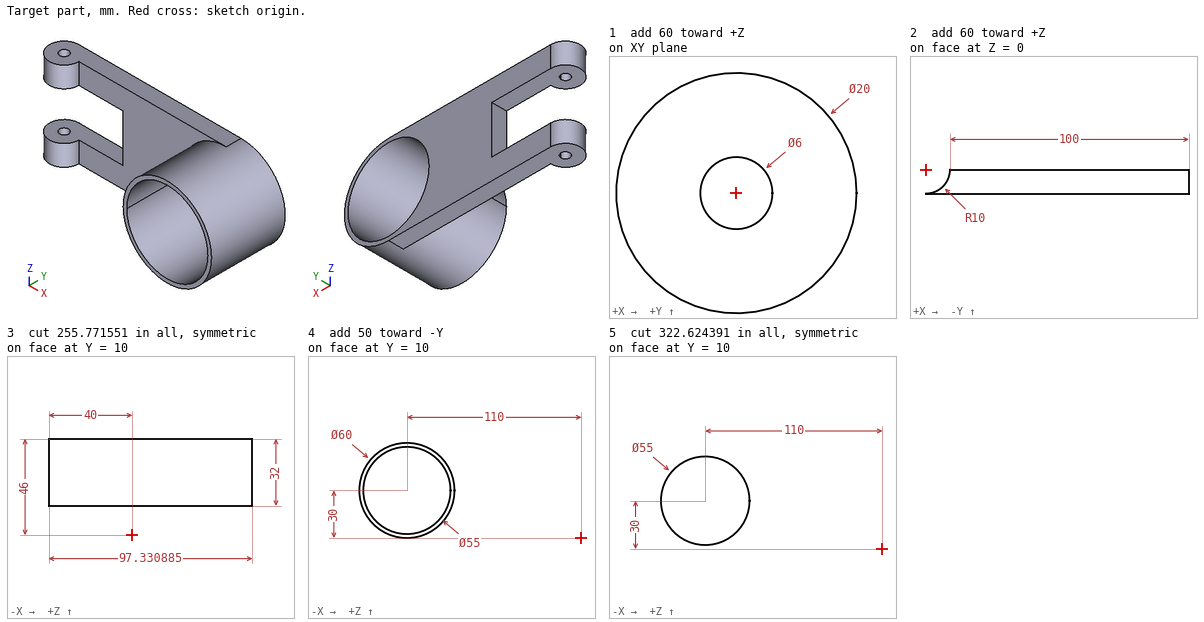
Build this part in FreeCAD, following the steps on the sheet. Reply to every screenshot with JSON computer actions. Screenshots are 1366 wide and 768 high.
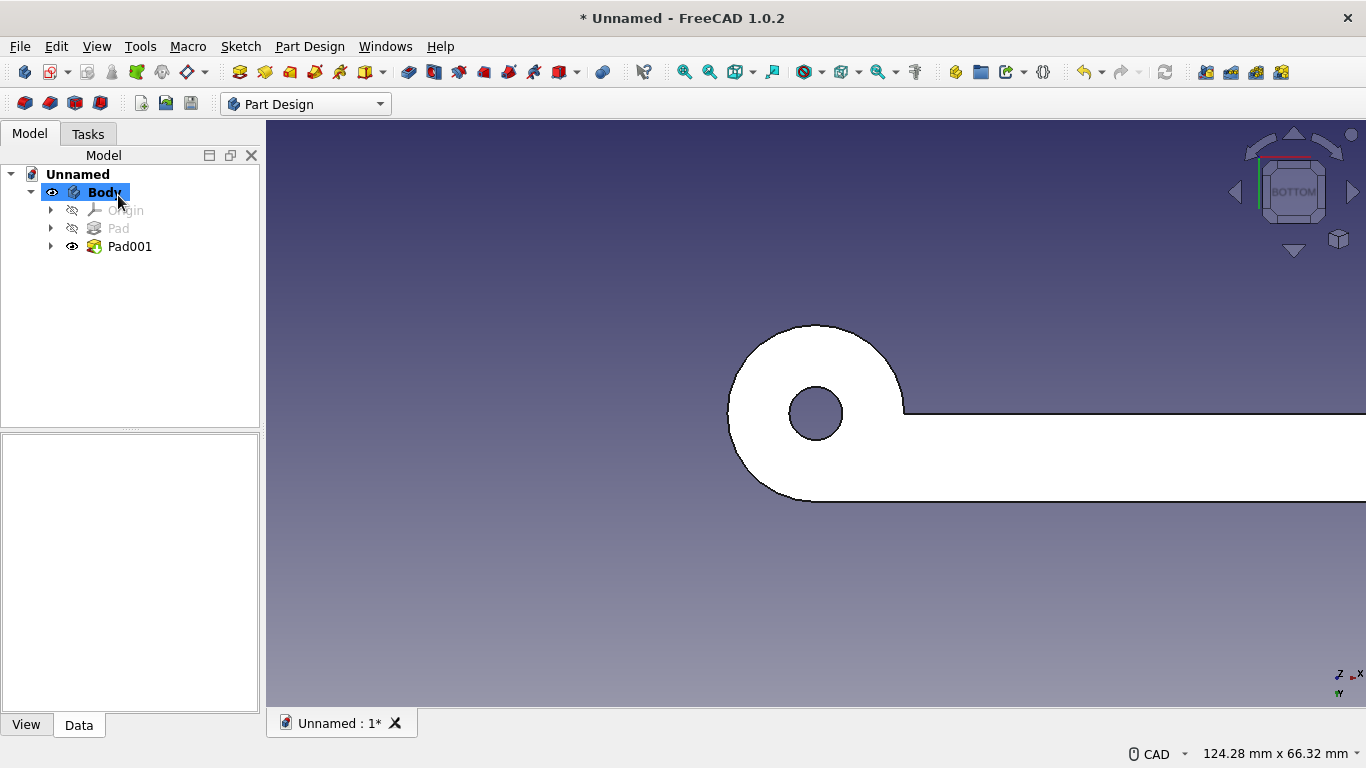
{"action": "left_click", "coordinate": [685, 72]}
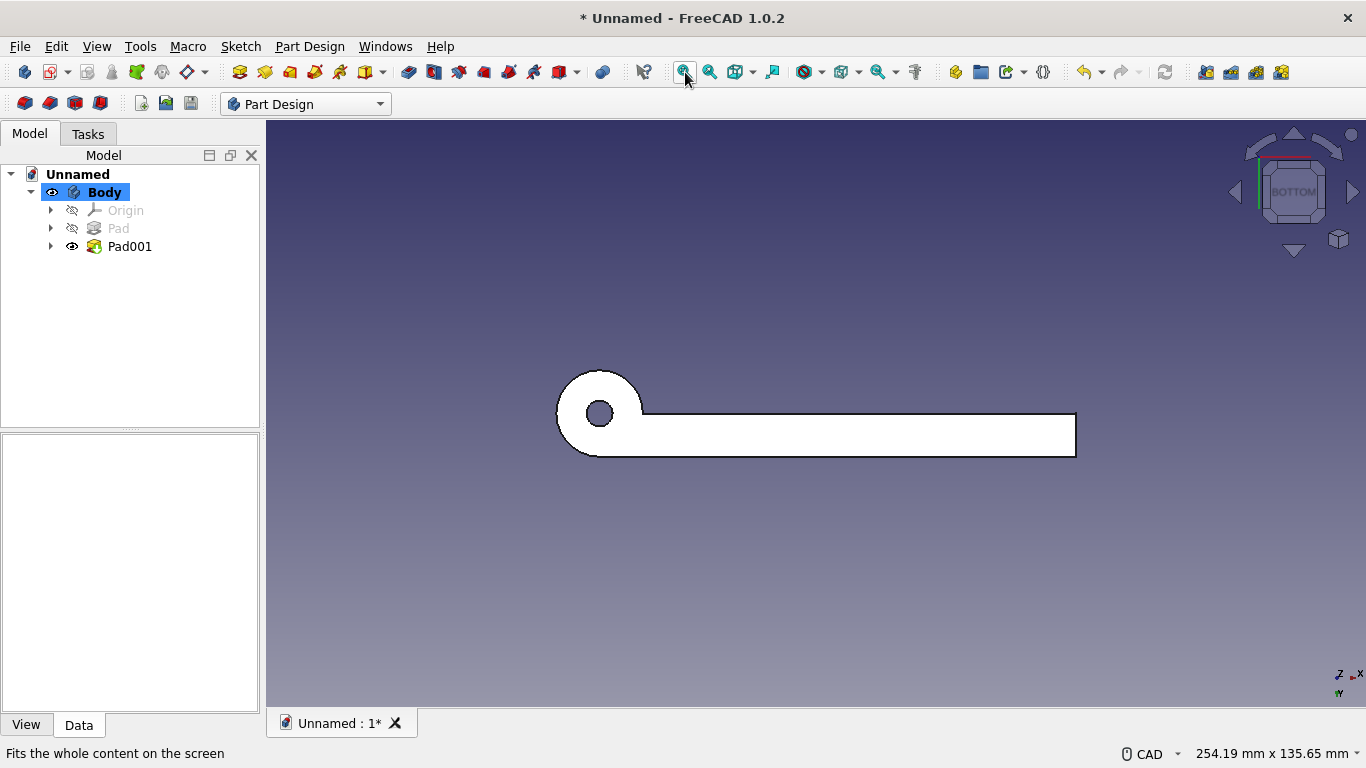
{"action": "key", "text": "4"}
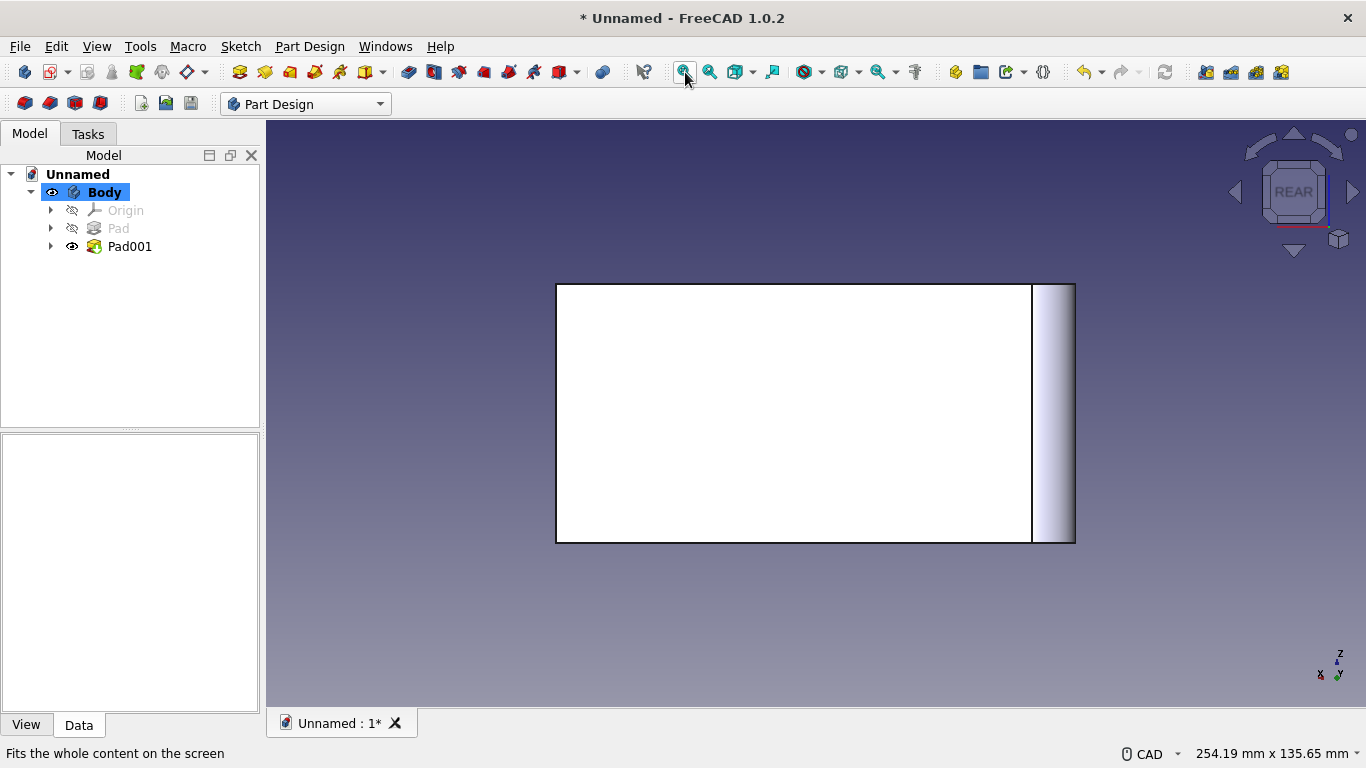
{"action": "left_click", "coordinate": [726, 412]}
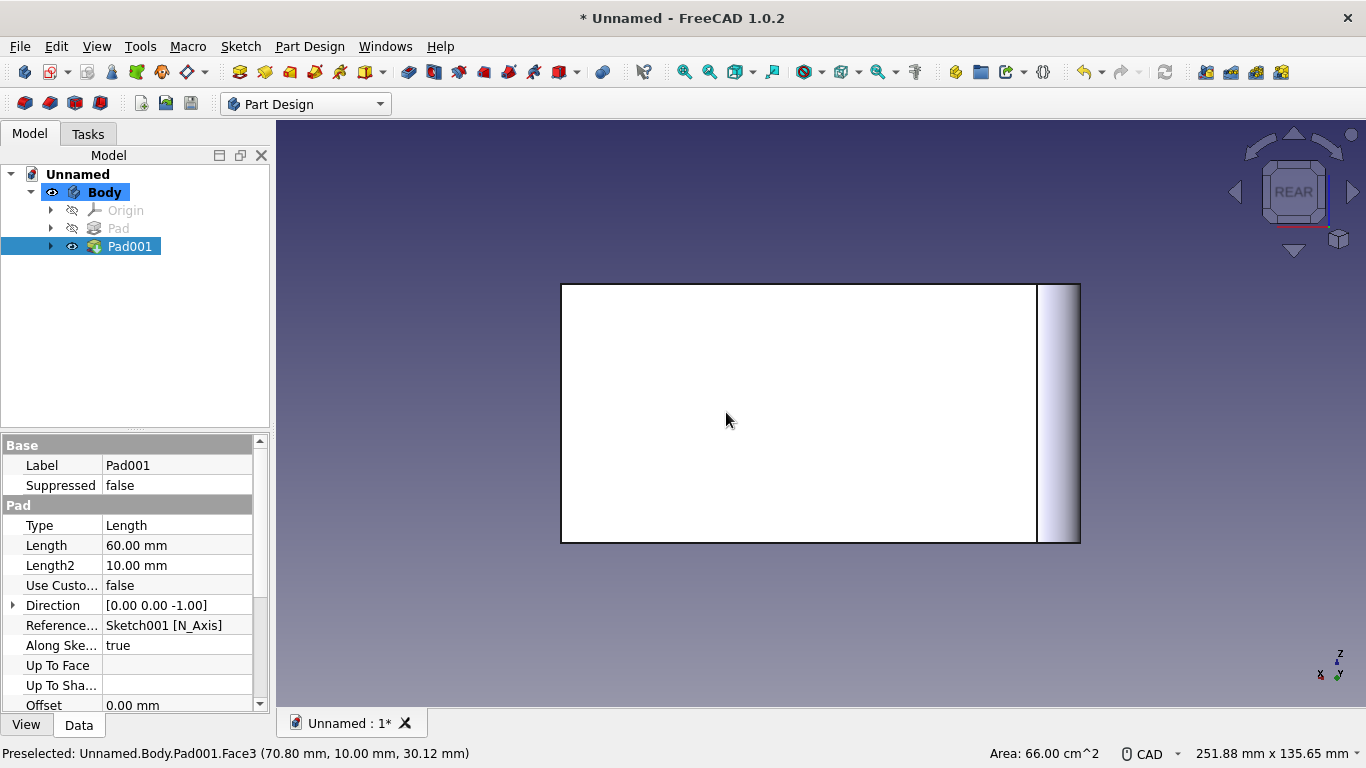
{"action": "left_click", "coordinate": [50, 72]}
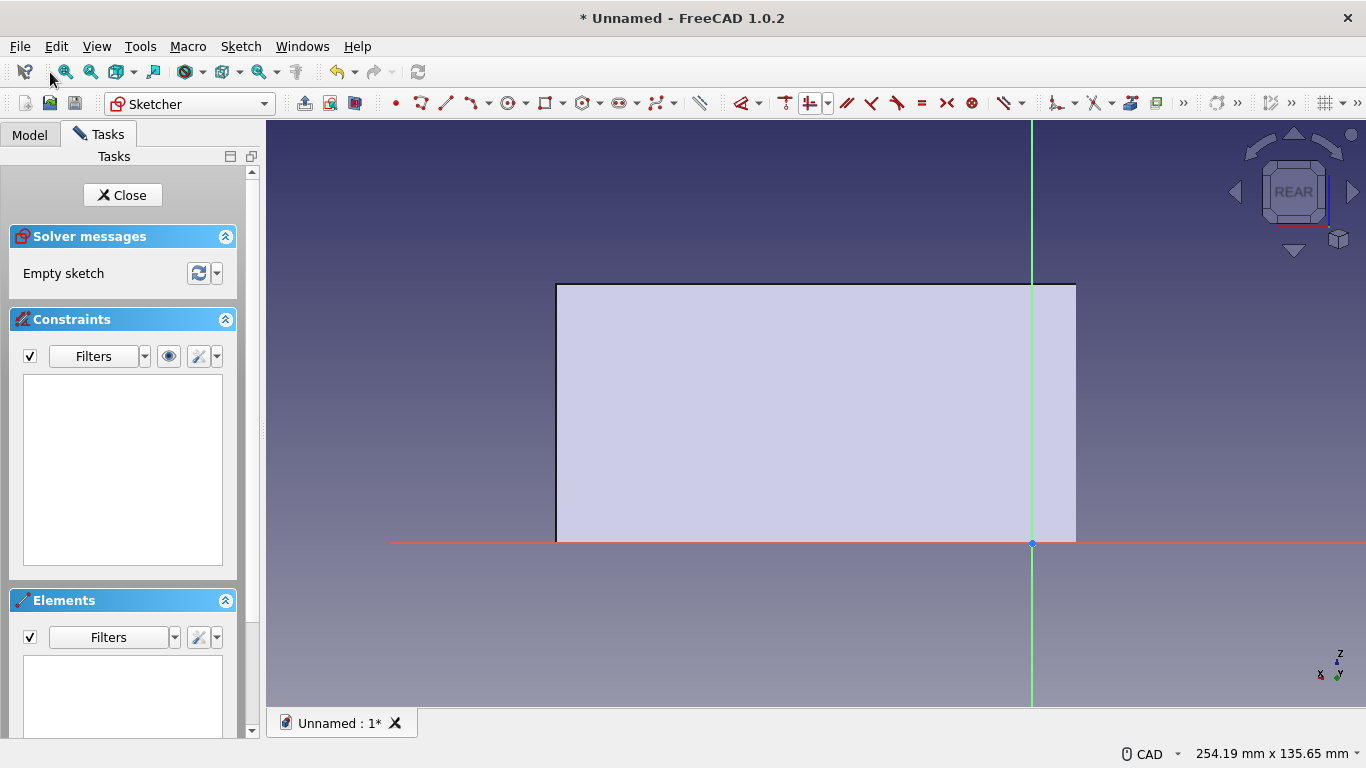
{"action": "scroll", "coordinate": [294, 277], "scroll_direction": "down", "scroll_amount": 1}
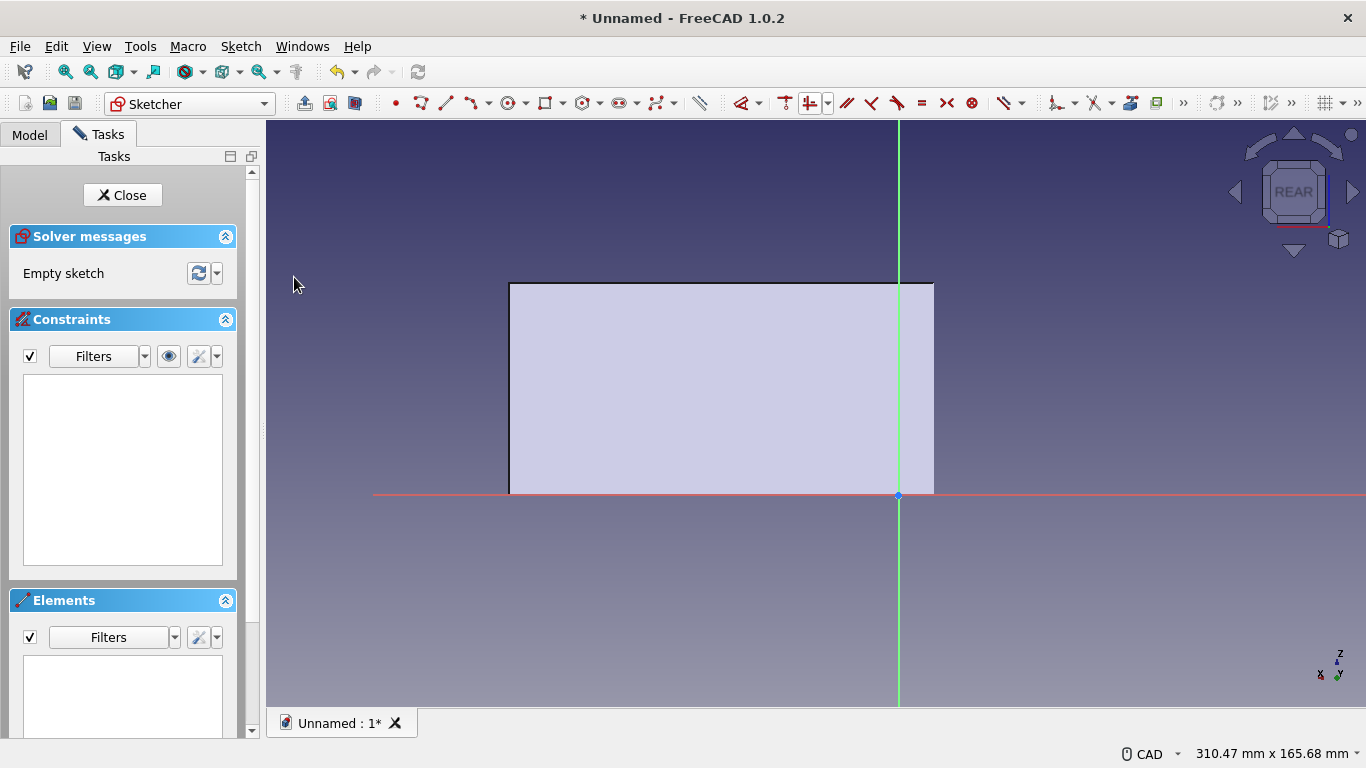
{"action": "scroll", "coordinate": [1150, 414], "scroll_direction": "up", "scroll_amount": 3}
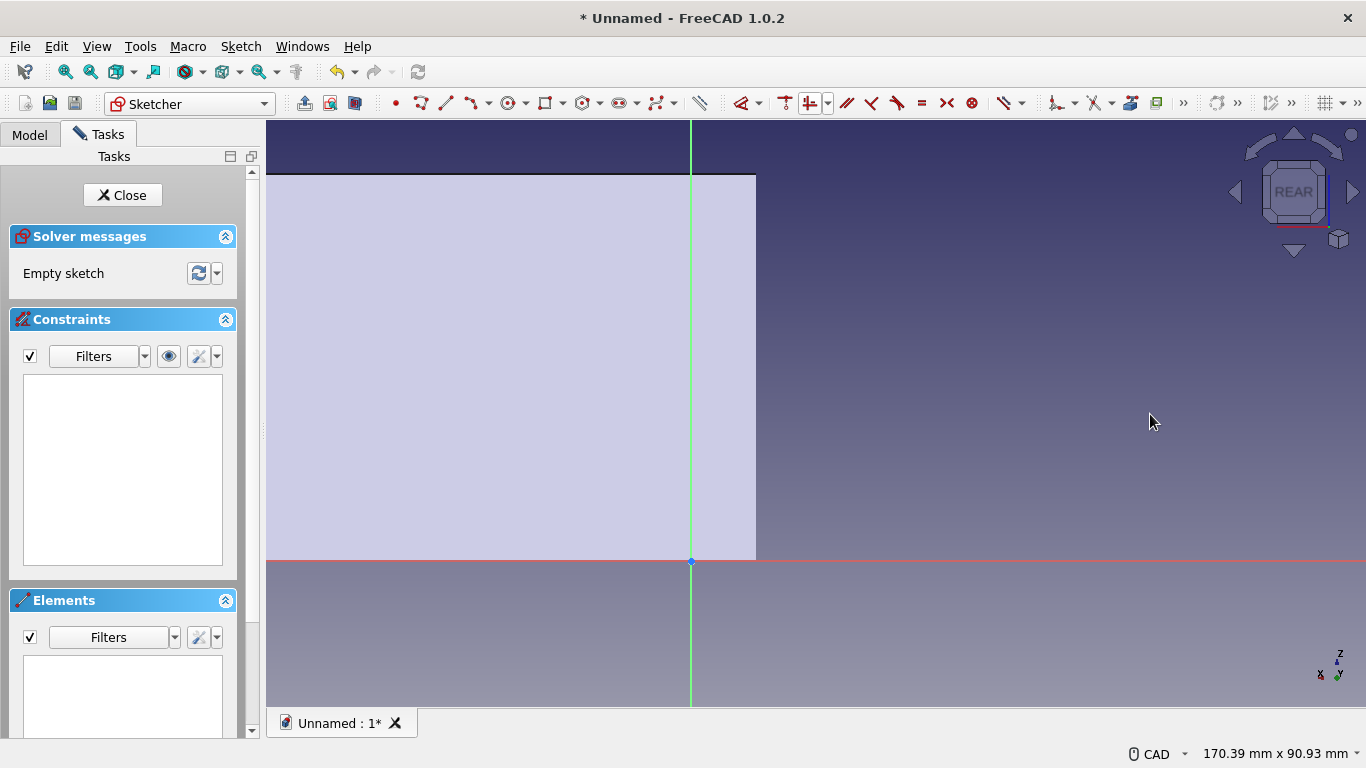
{"action": "left_click", "coordinate": [544, 104]}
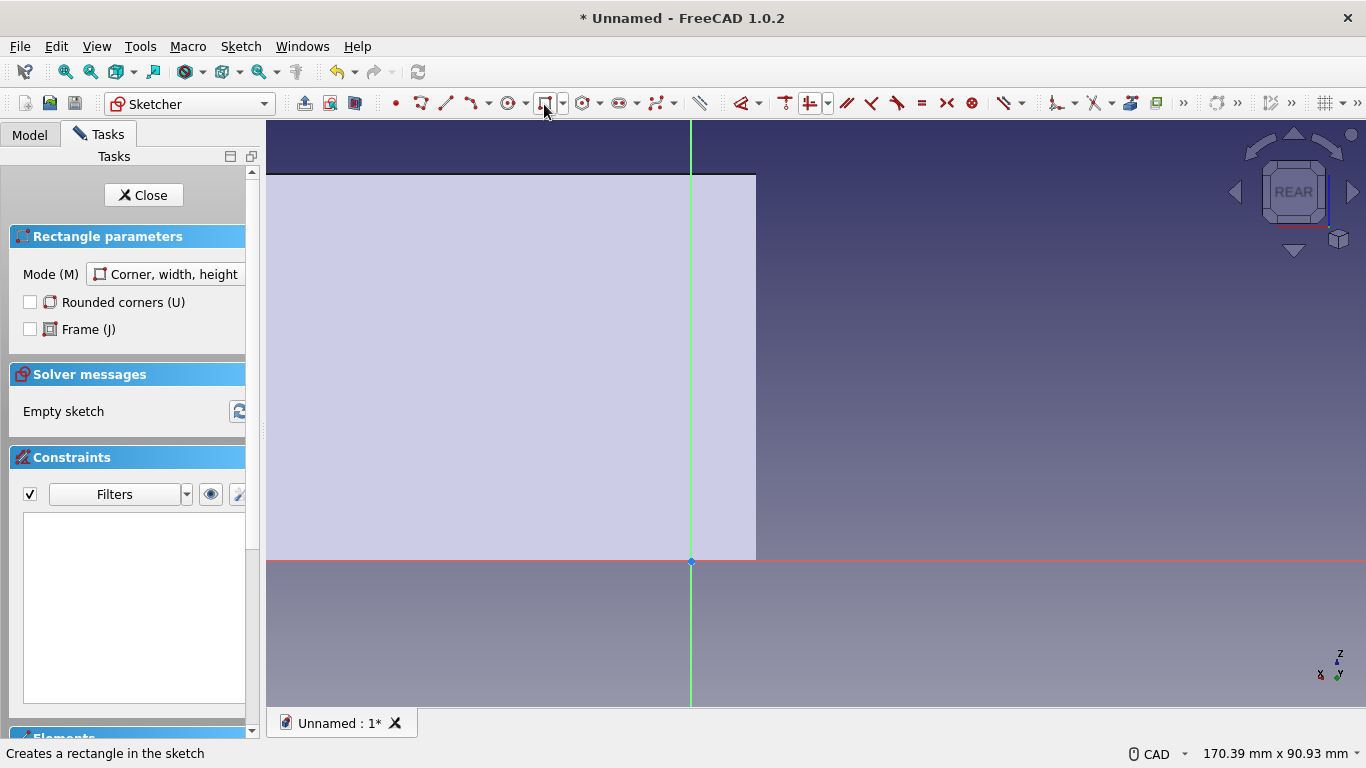
{"action": "left_click", "coordinate": [433, 264]}
{"action": "mouse_move", "coordinate": [1061, 471]}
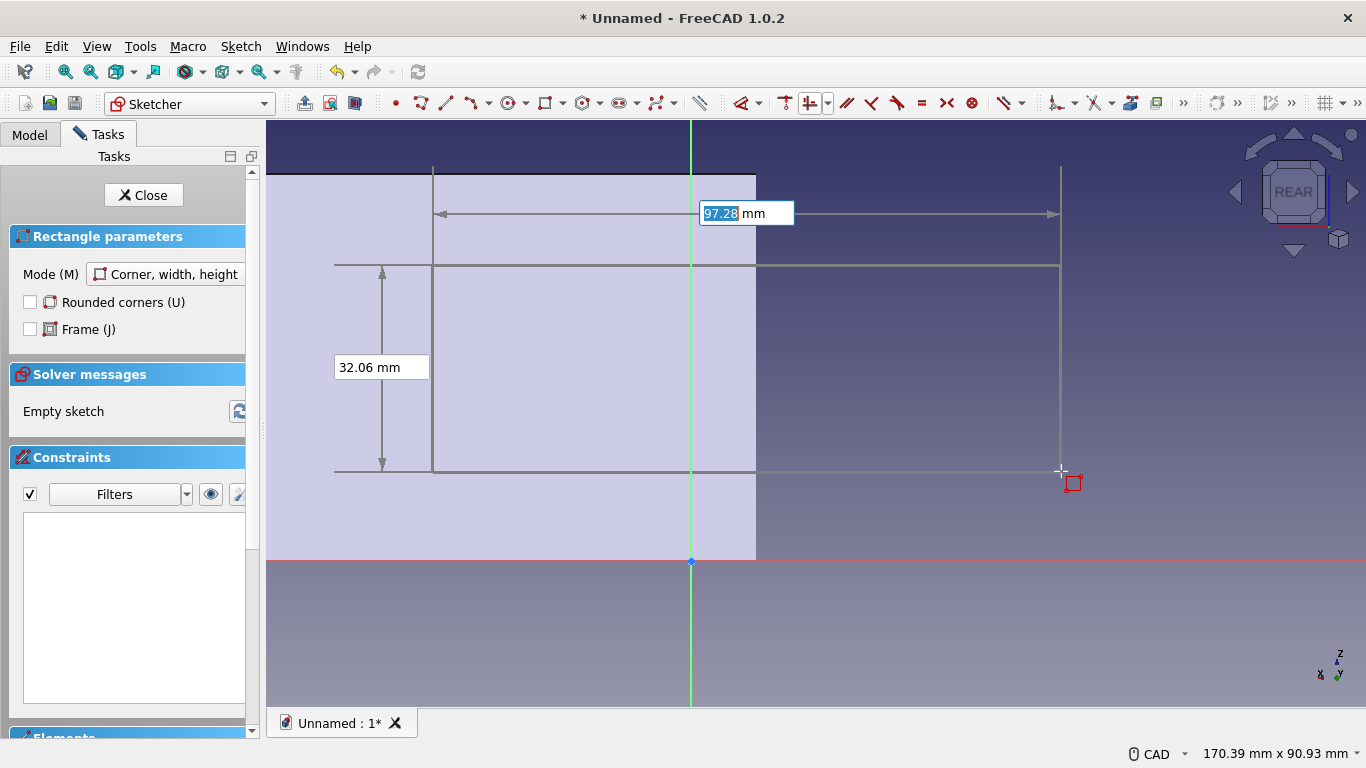
{"action": "type", "text": "97.330885"}
{"action": "key", "text": "Tab"}
{"action": "type", "text": "32"}
{"action": "key", "text": "Return"}
{"action": "key", "text": "Escape"}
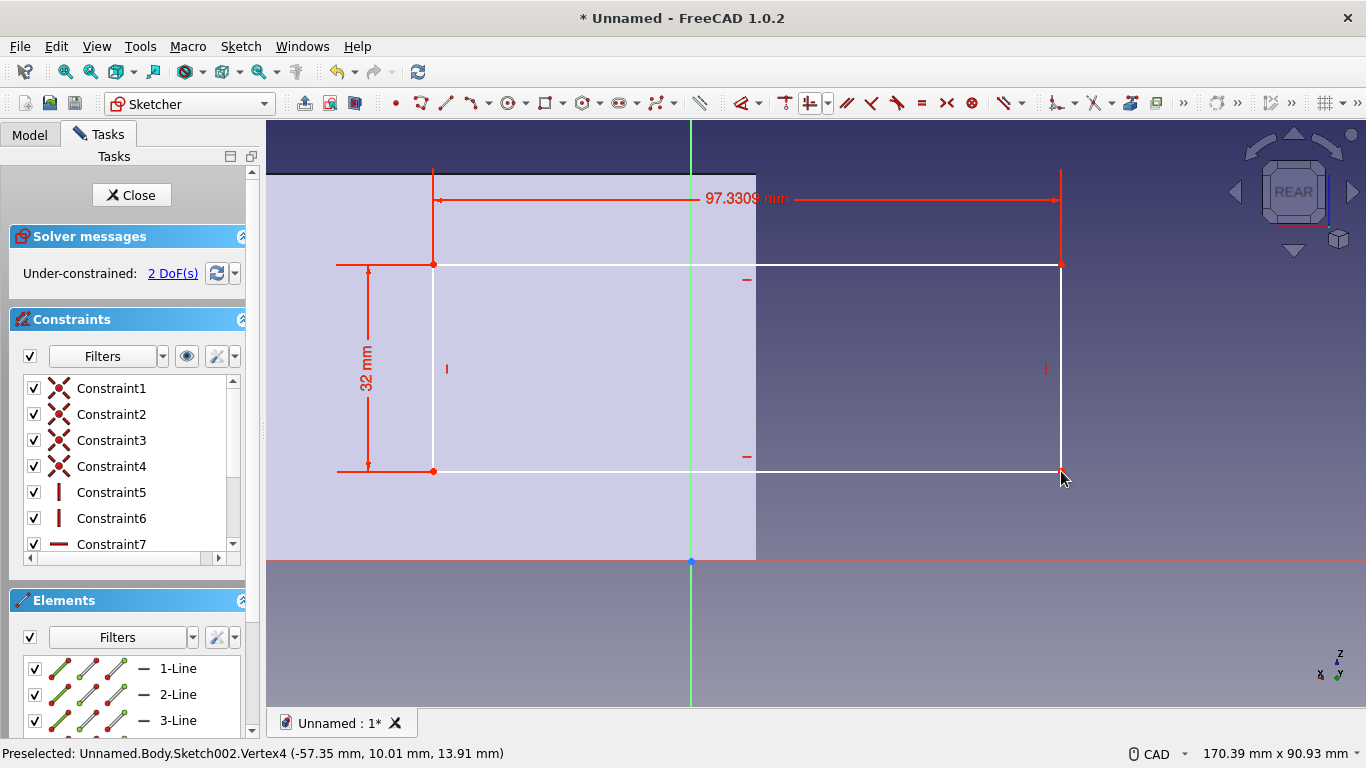
{"action": "left_click", "coordinate": [740, 104]}